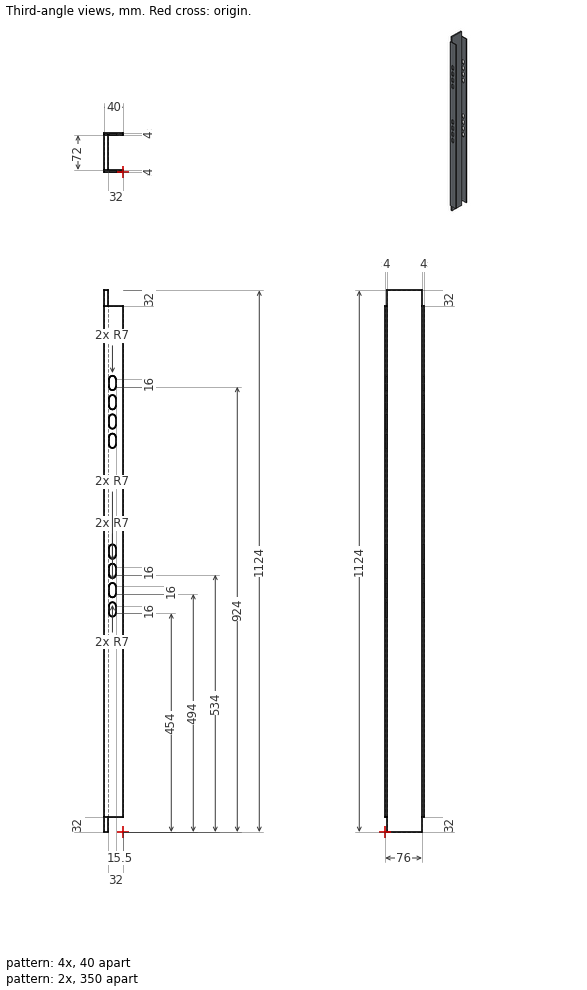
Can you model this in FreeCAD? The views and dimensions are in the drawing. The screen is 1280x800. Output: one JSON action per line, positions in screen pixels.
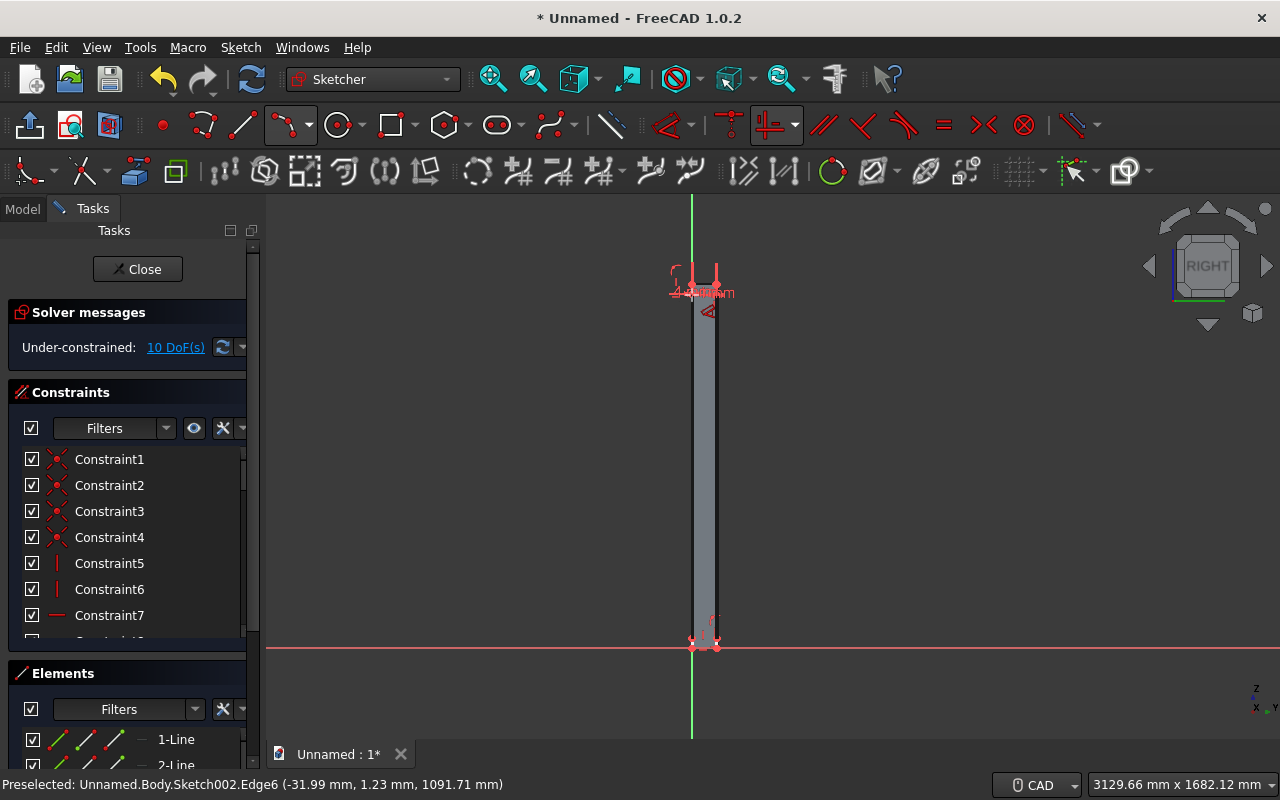
{"action": "scroll", "coordinate": [717, 648], "scroll_direction": "up", "scroll_amount": 18}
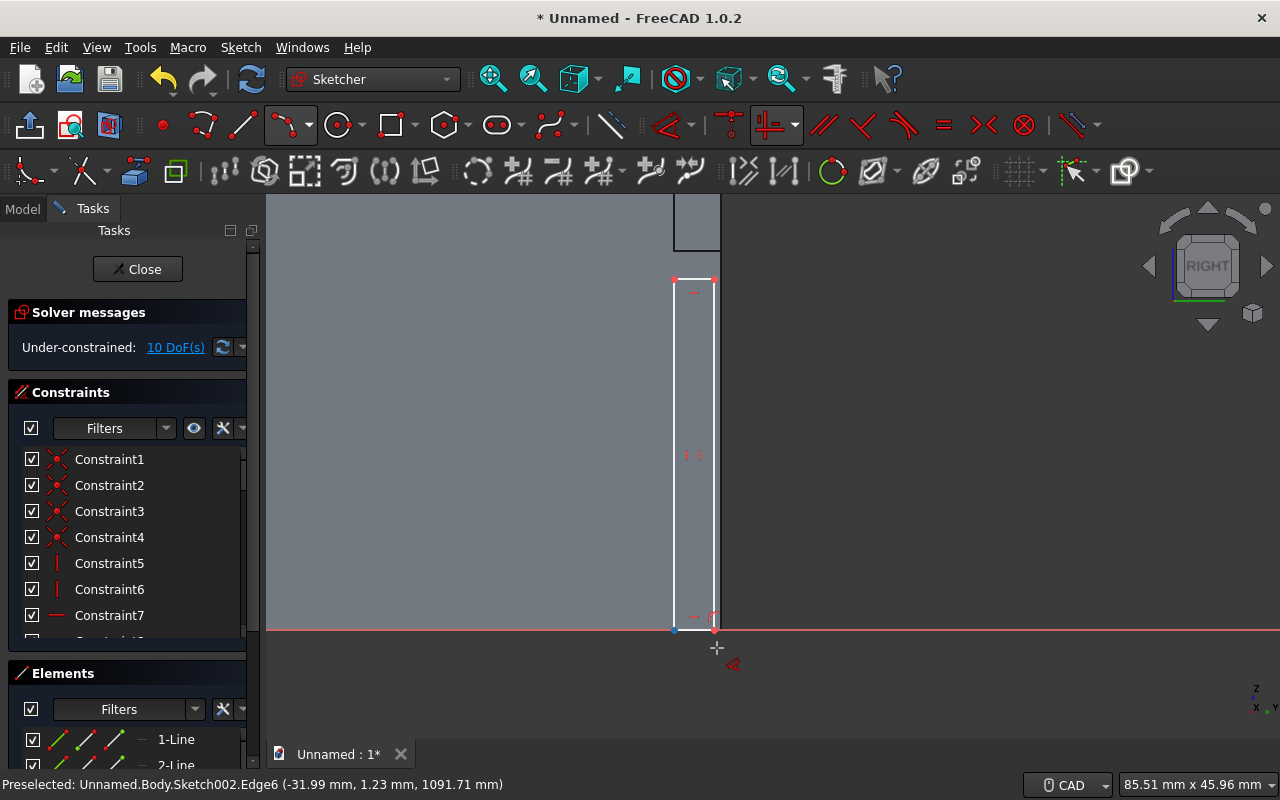
{"action": "left_click", "coordinate": [686, 630]}
{"action": "left_click", "coordinate": [694, 664]}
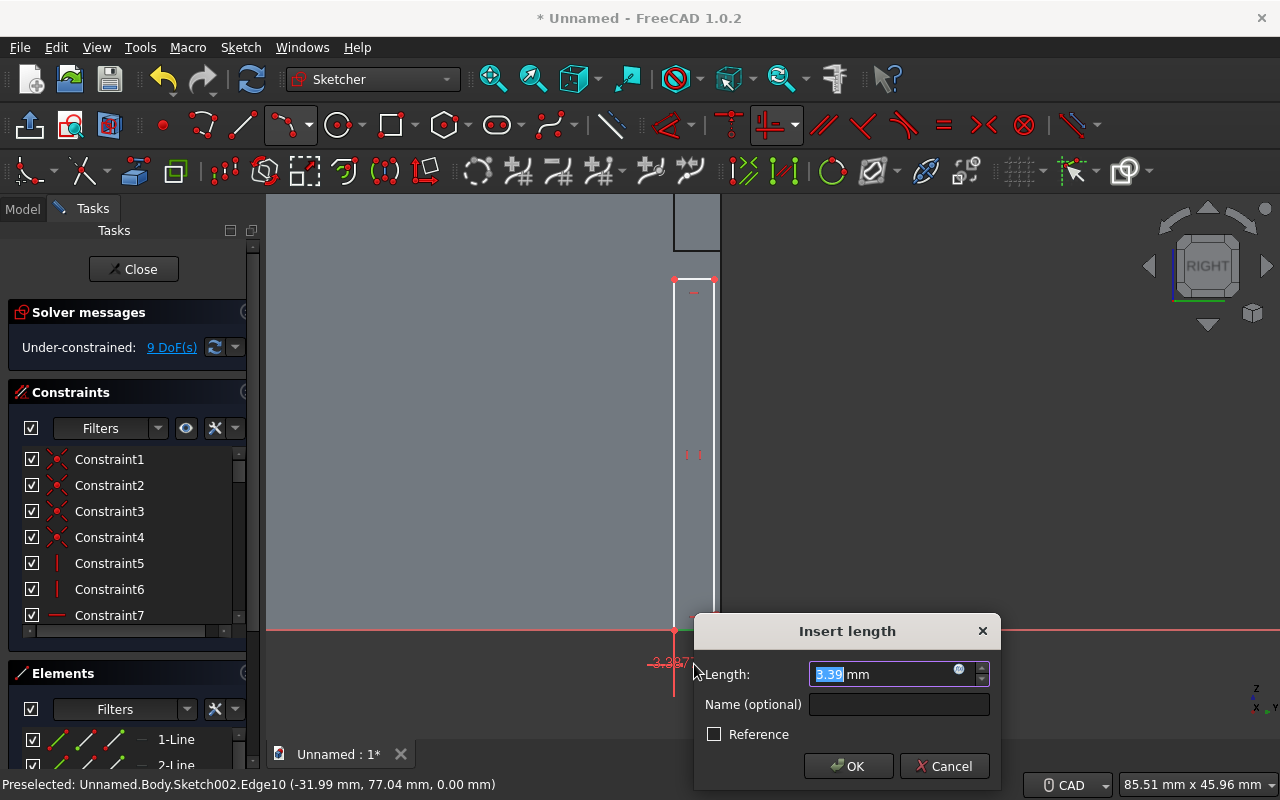
{"action": "type", "text": "4"}
{"action": "key", "text": "Return"}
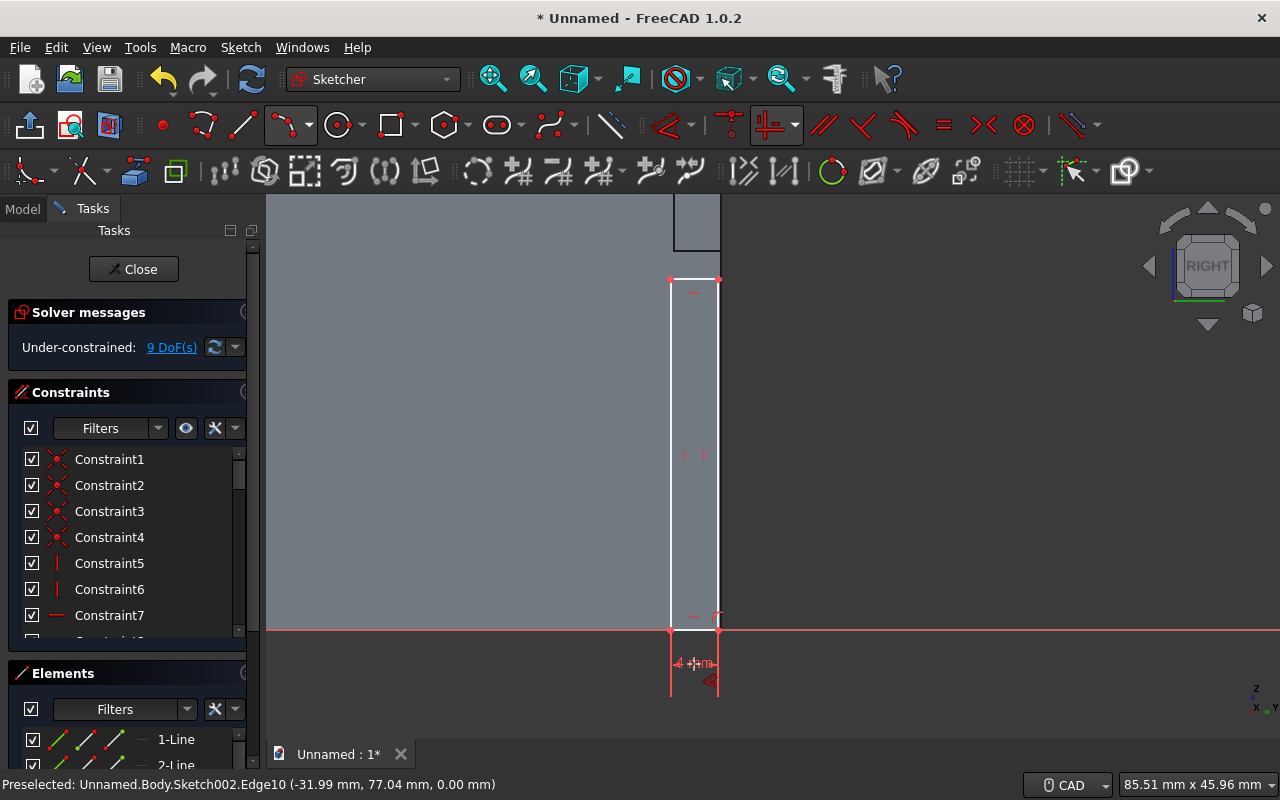
{"action": "scroll", "coordinate": [717, 649], "scroll_direction": "down", "scroll_amount": 18}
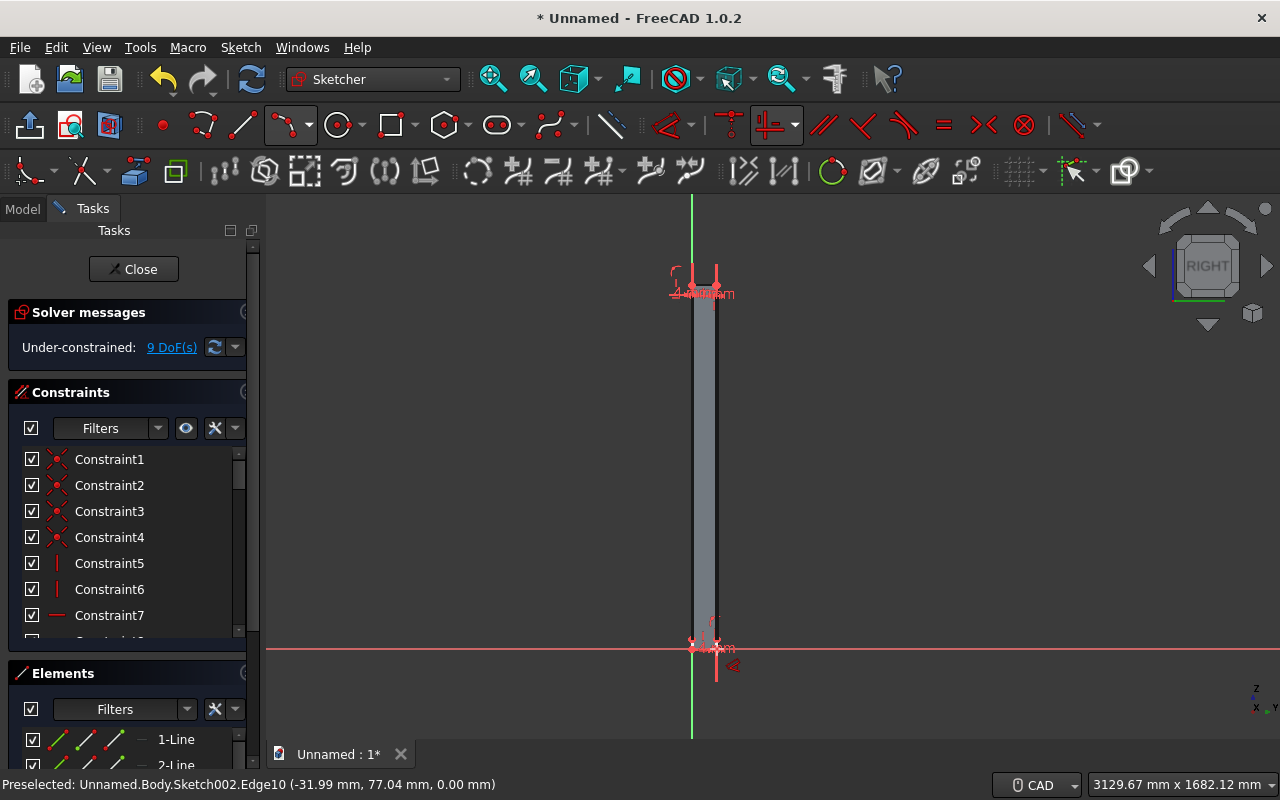
{"action": "scroll", "coordinate": [692, 649], "scroll_direction": "up", "scroll_amount": 18}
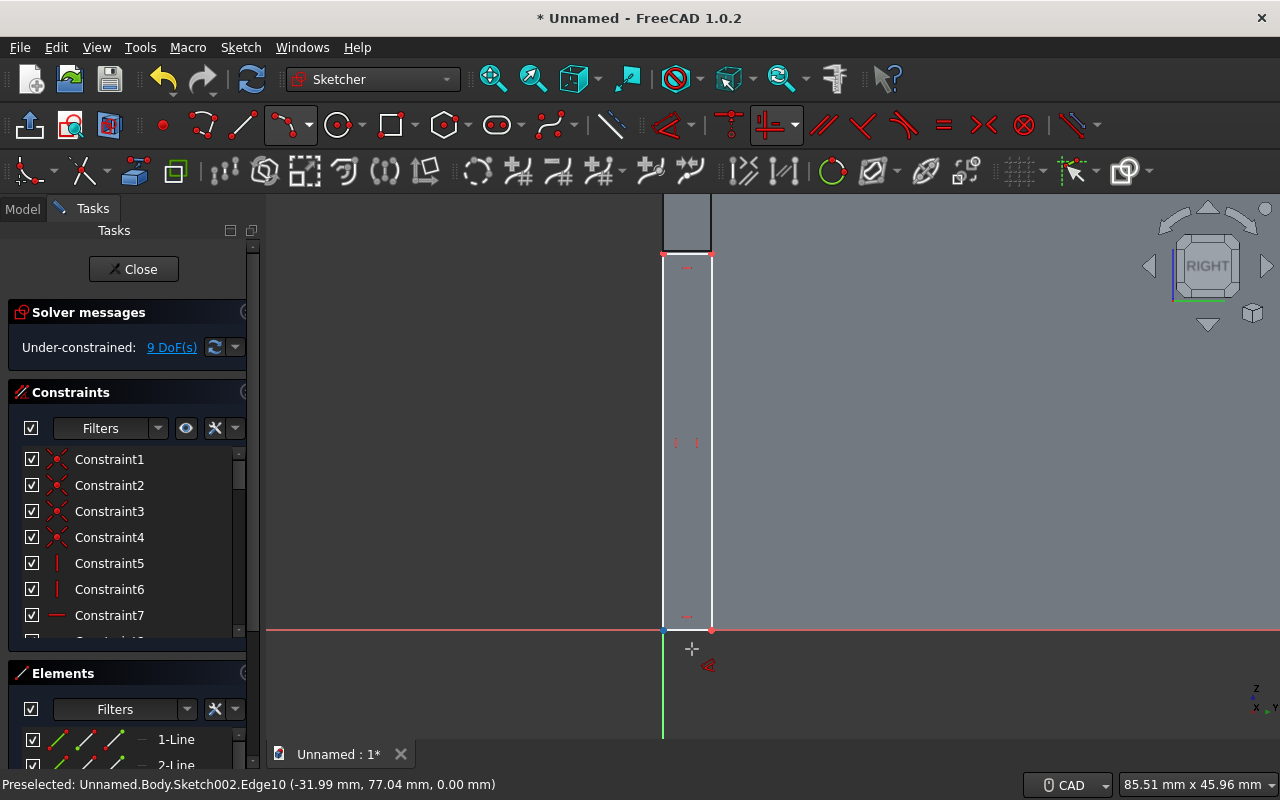
{"action": "left_click", "coordinate": [678, 630]}
{"action": "left_click", "coordinate": [687, 664]}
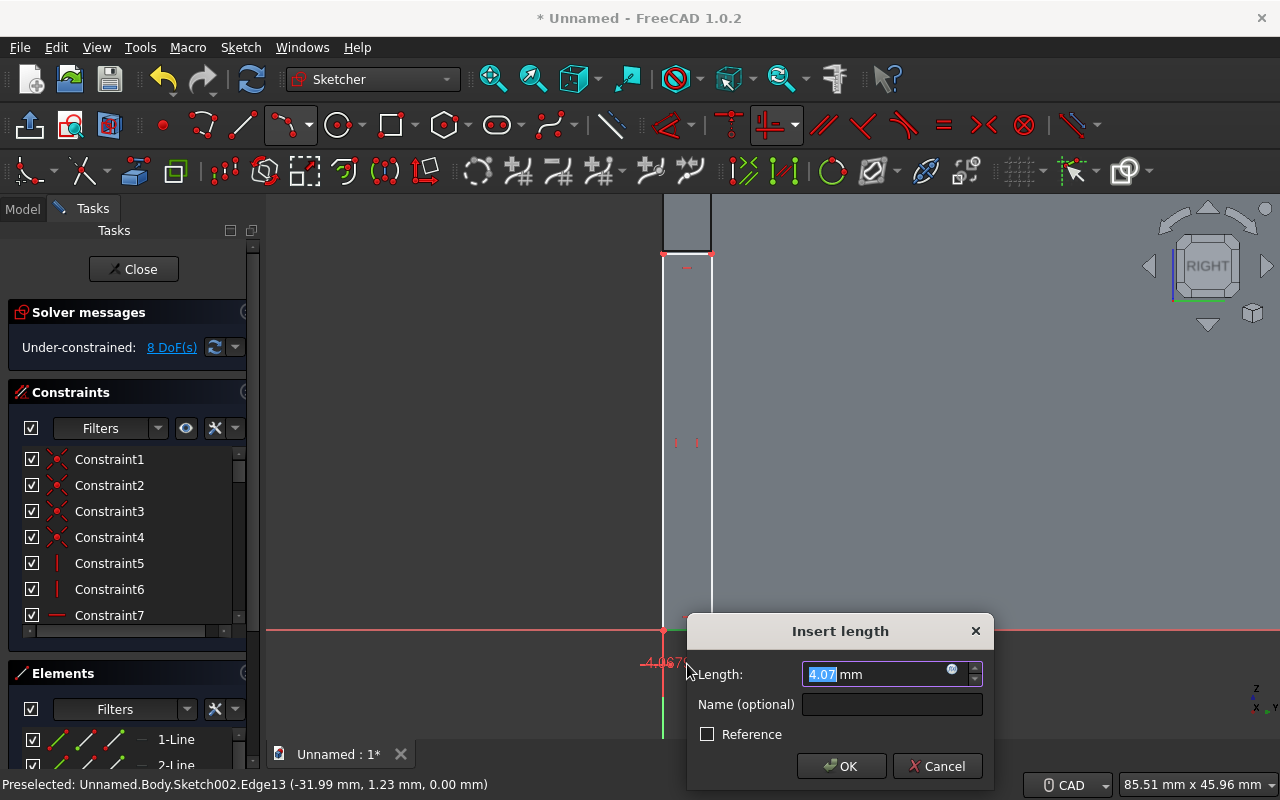
{"action": "type", "text": "4"}
{"action": "key", "text": "Return"}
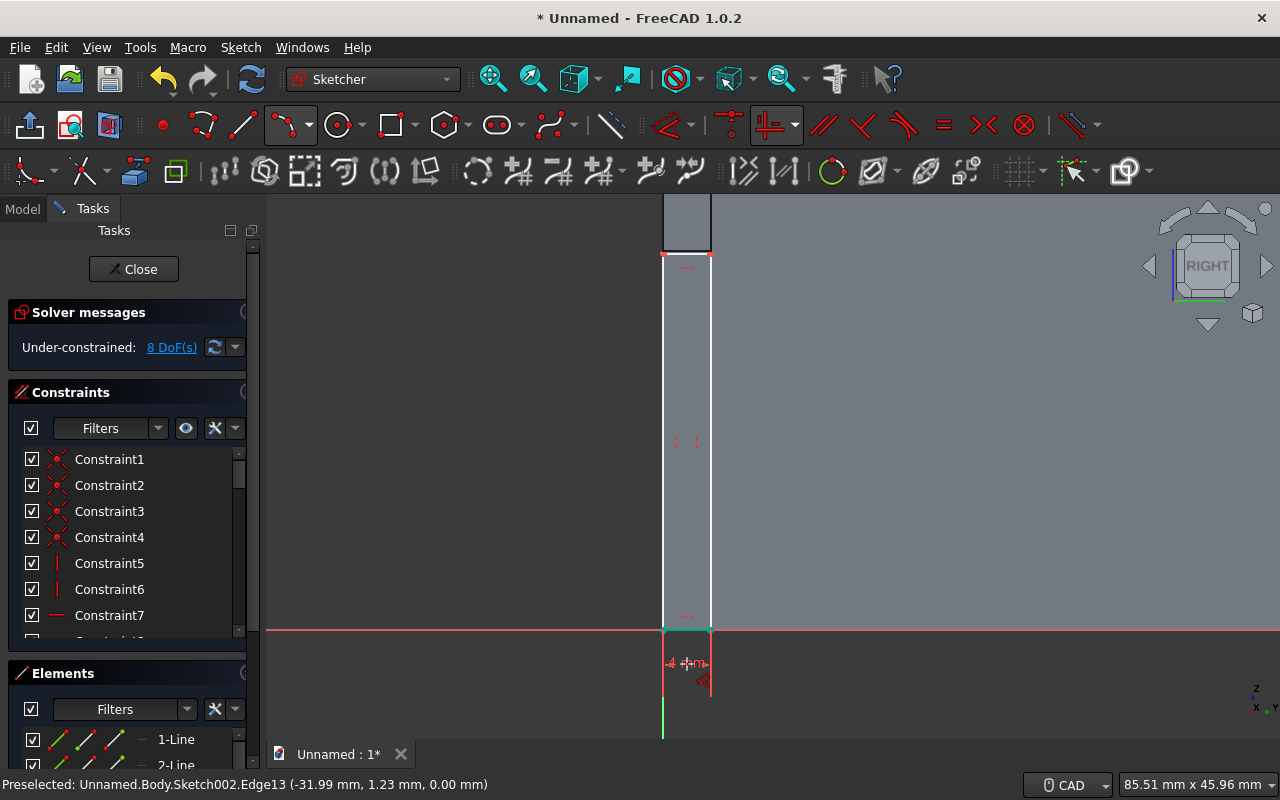
{"action": "scroll", "coordinate": [692, 649], "scroll_direction": "down", "scroll_amount": 18}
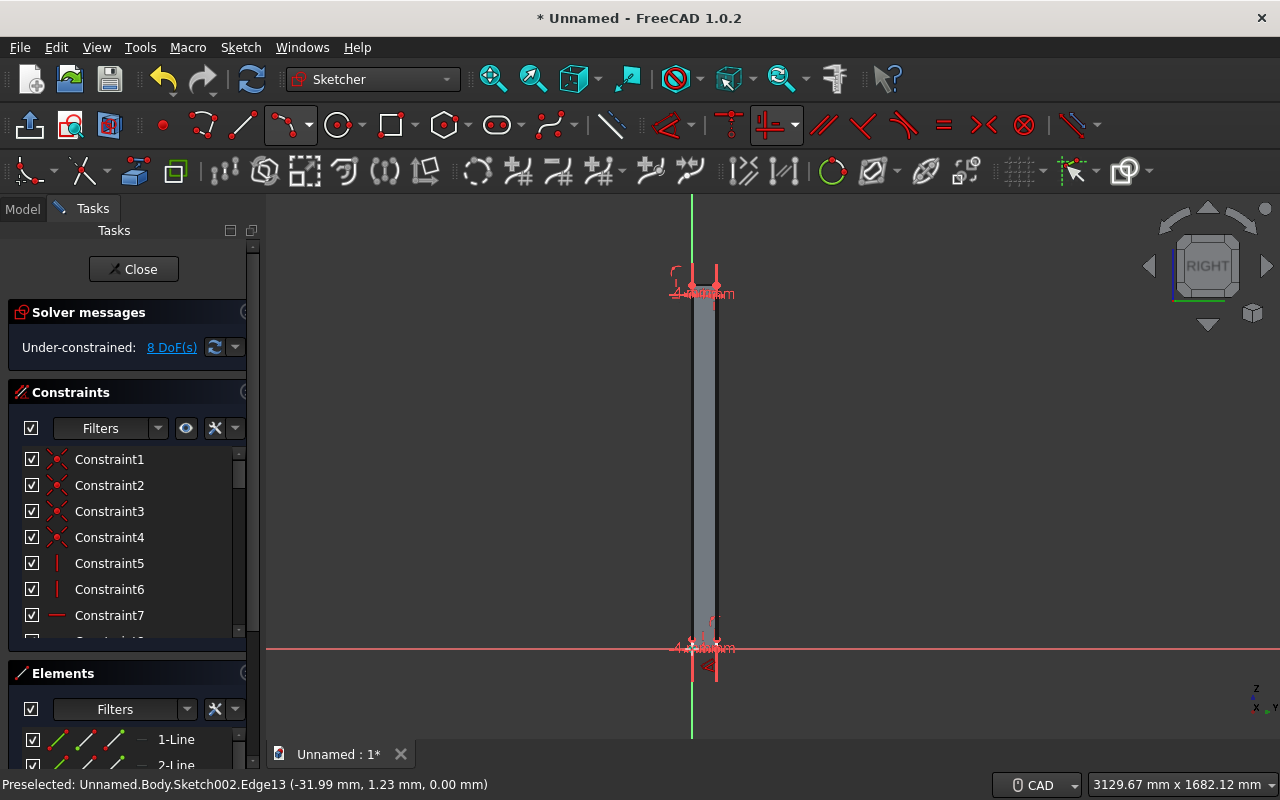
{"action": "scroll", "coordinate": [716, 289], "scroll_direction": "up", "scroll_amount": 12}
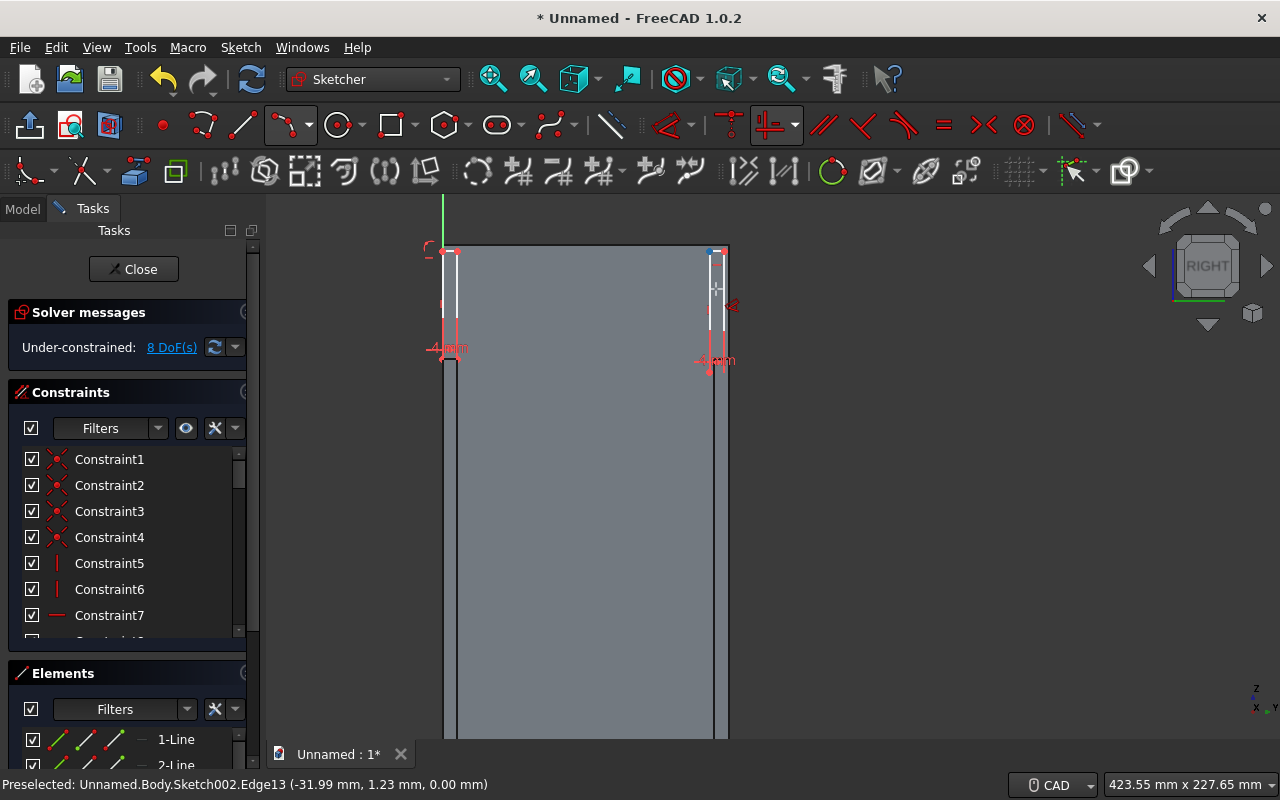
{"action": "left_click", "coordinate": [710, 287]}
{"action": "left_click", "coordinate": [744, 312]}